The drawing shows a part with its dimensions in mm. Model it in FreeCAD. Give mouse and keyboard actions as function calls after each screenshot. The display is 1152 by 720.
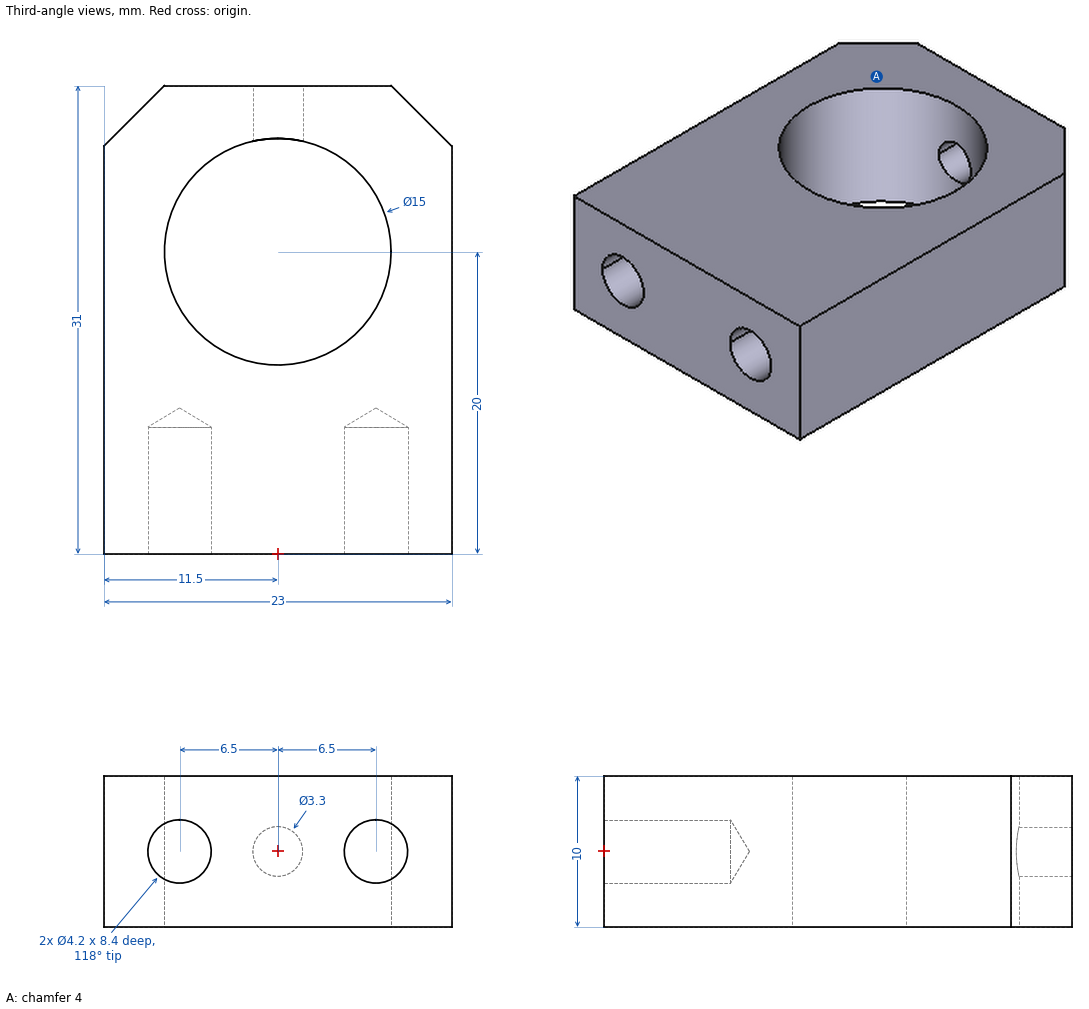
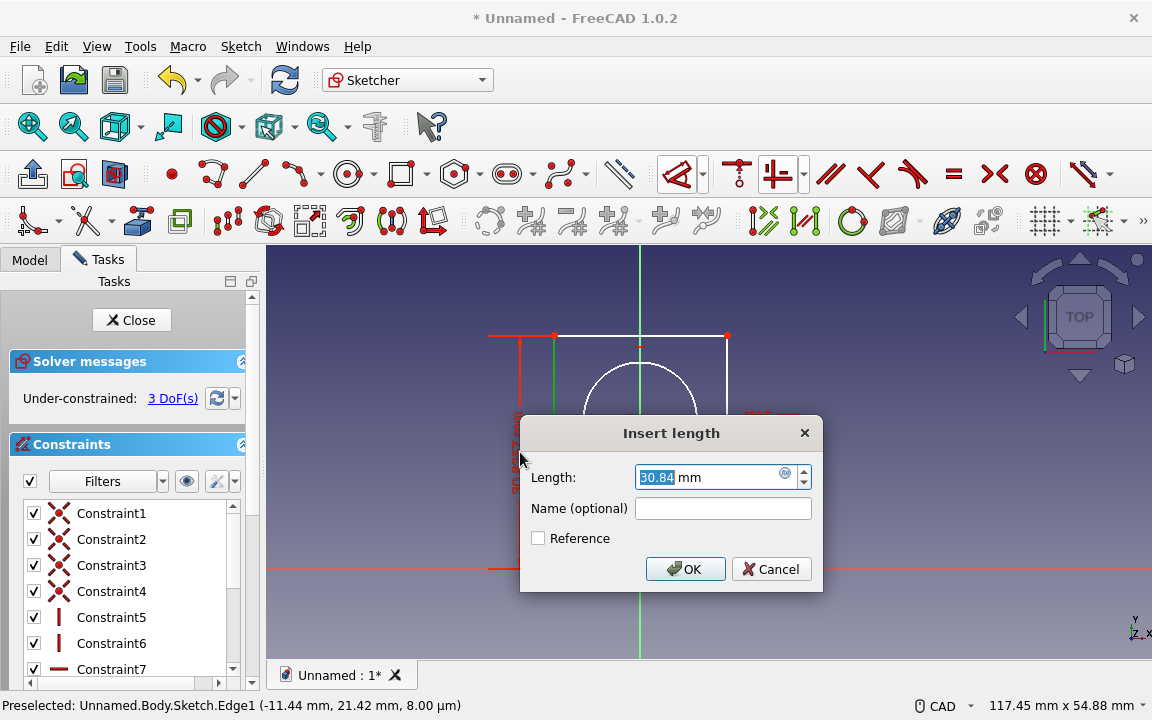
text(31)
key(Return)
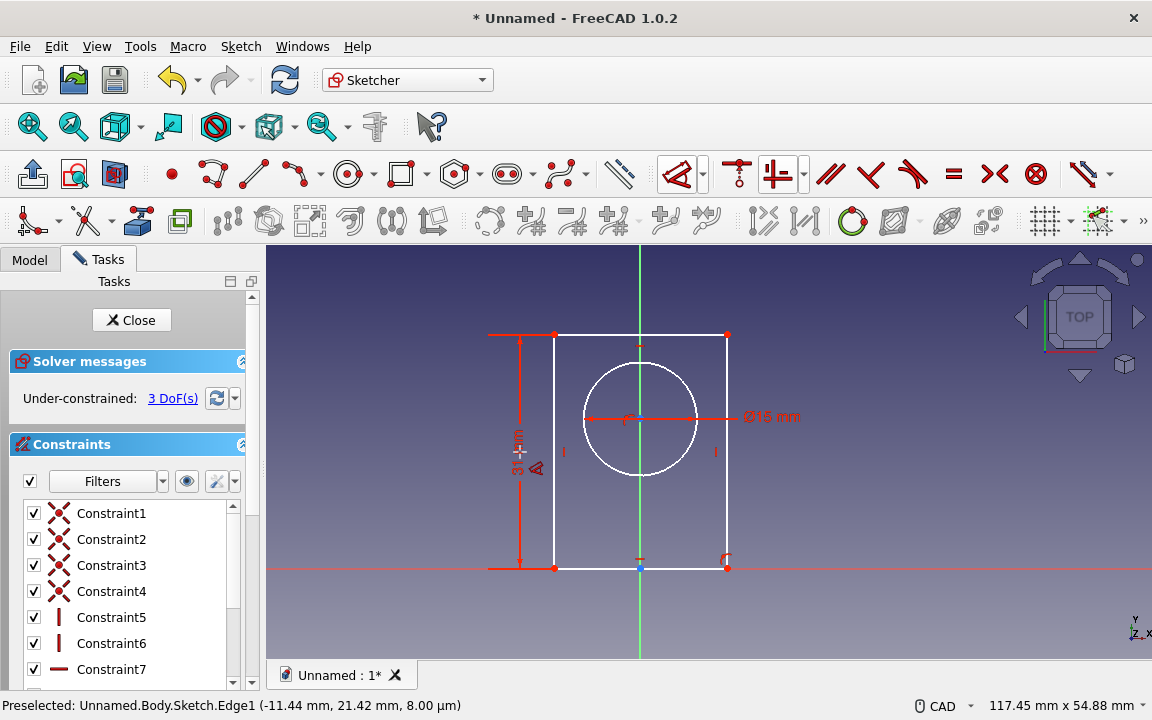
click(606, 569)
click(601, 603)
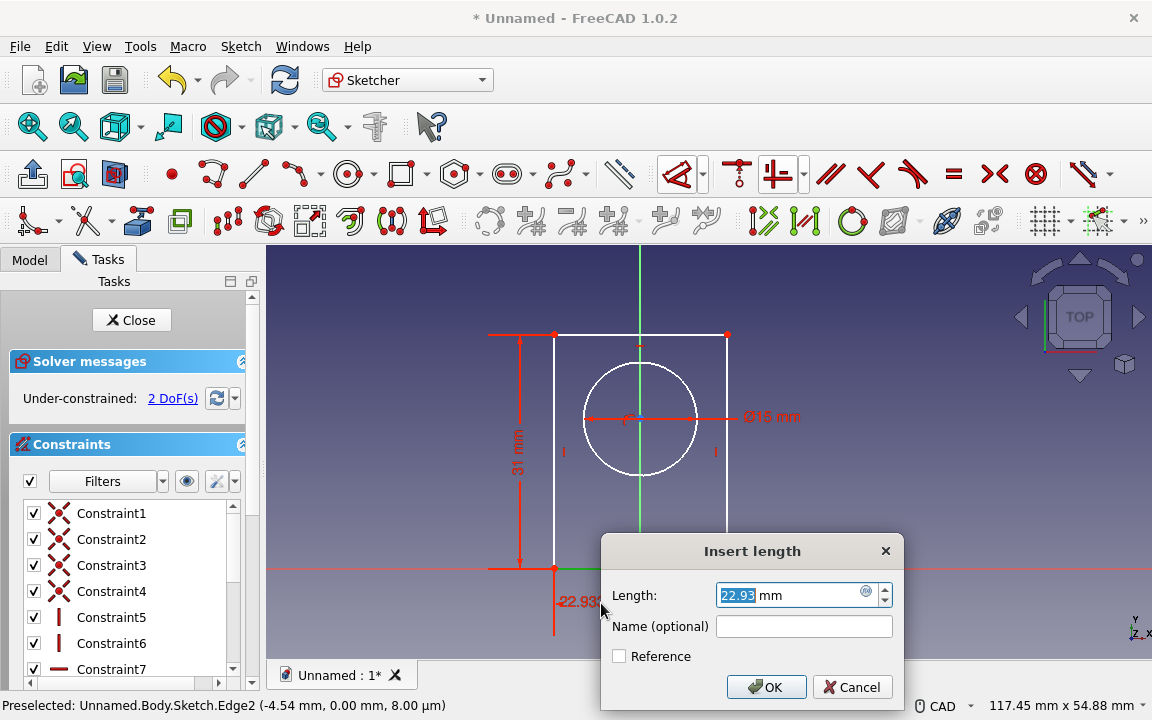
text(23)
key(Return)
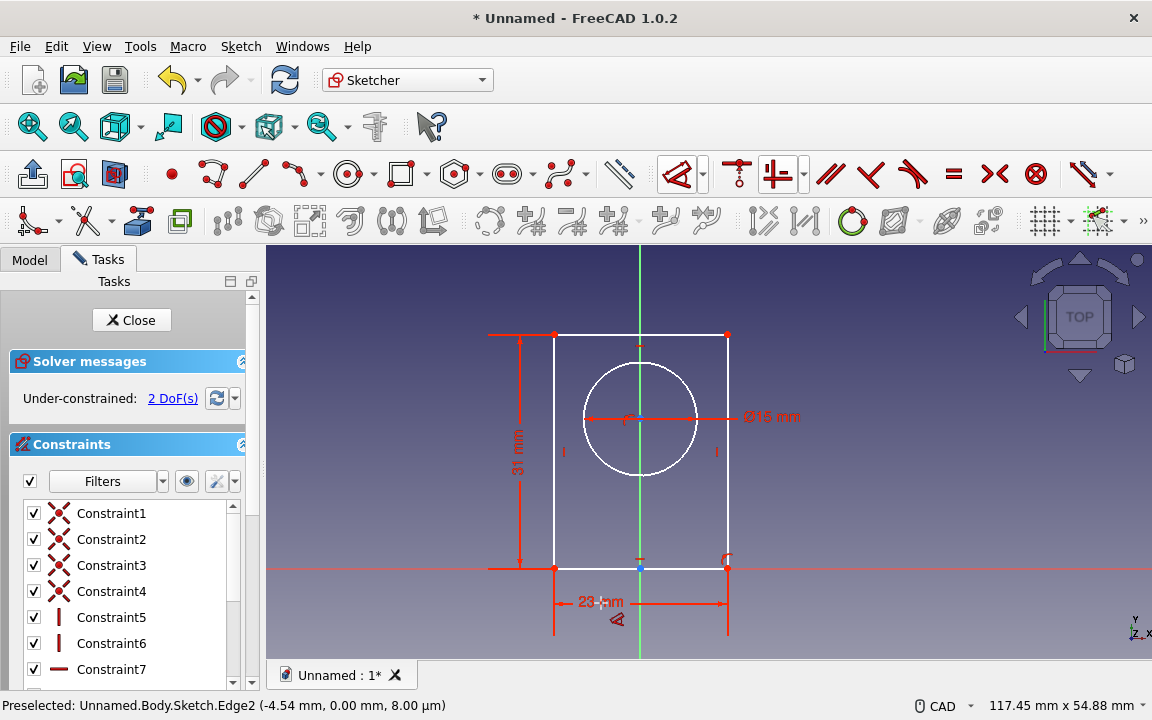
click(640, 419)
click(674, 494)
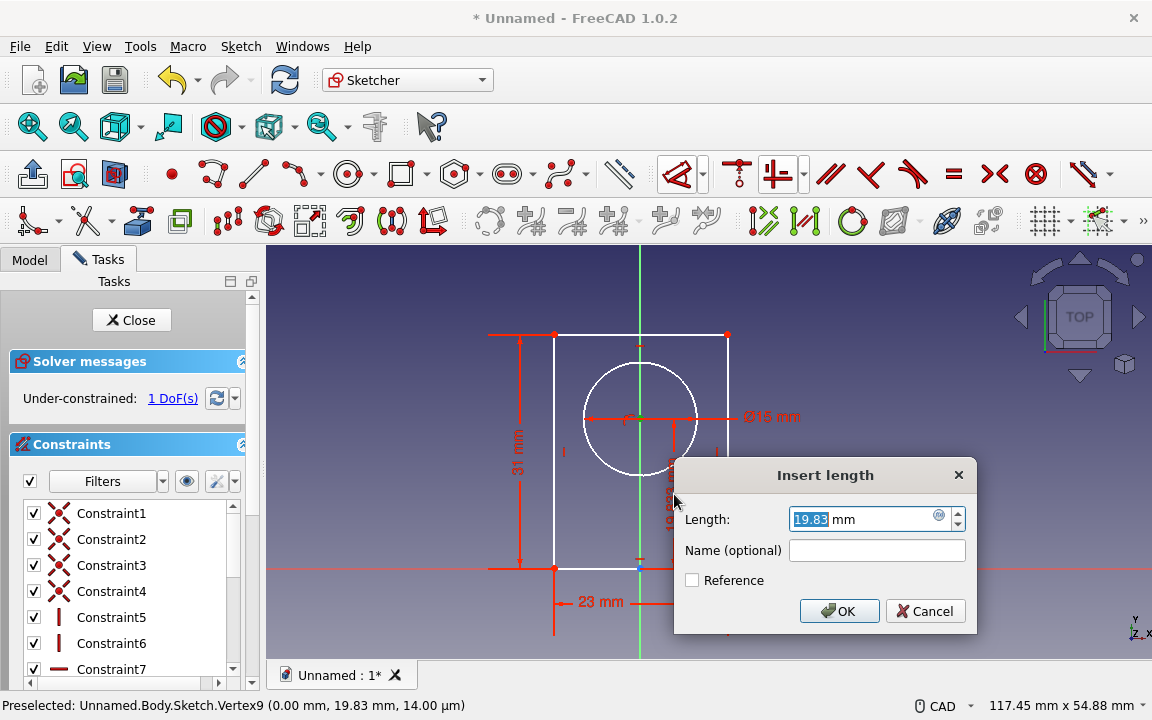
text(20)
key(Return)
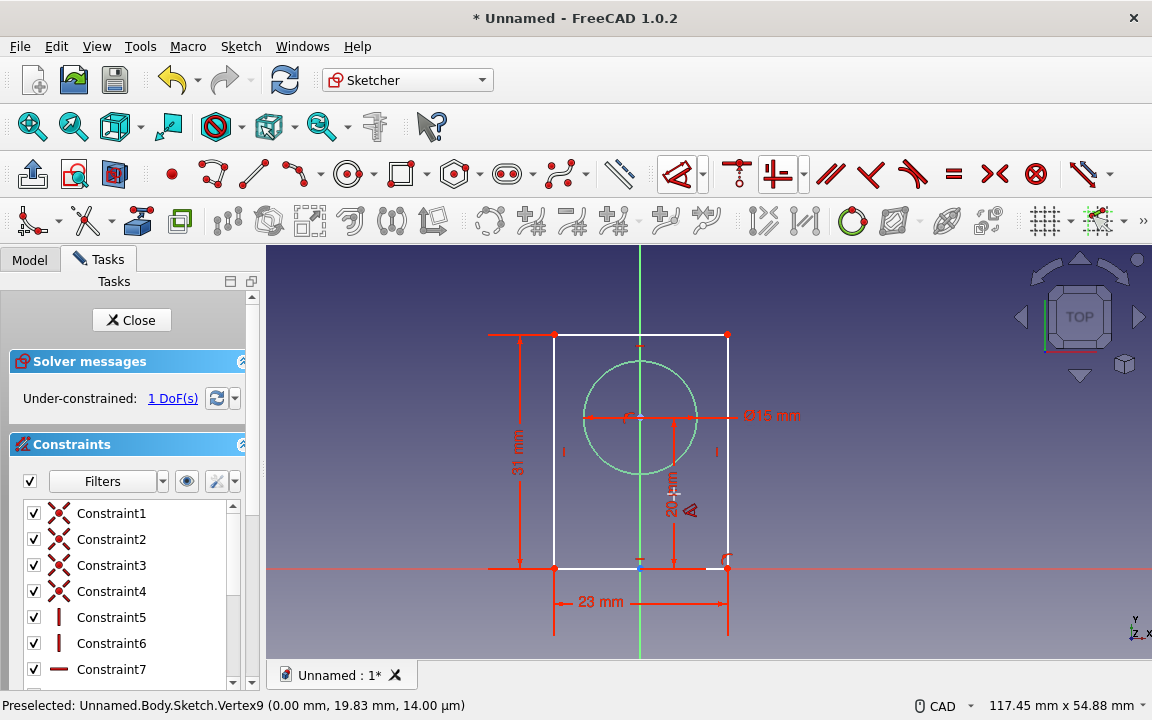
click(554, 335)
click(597, 301)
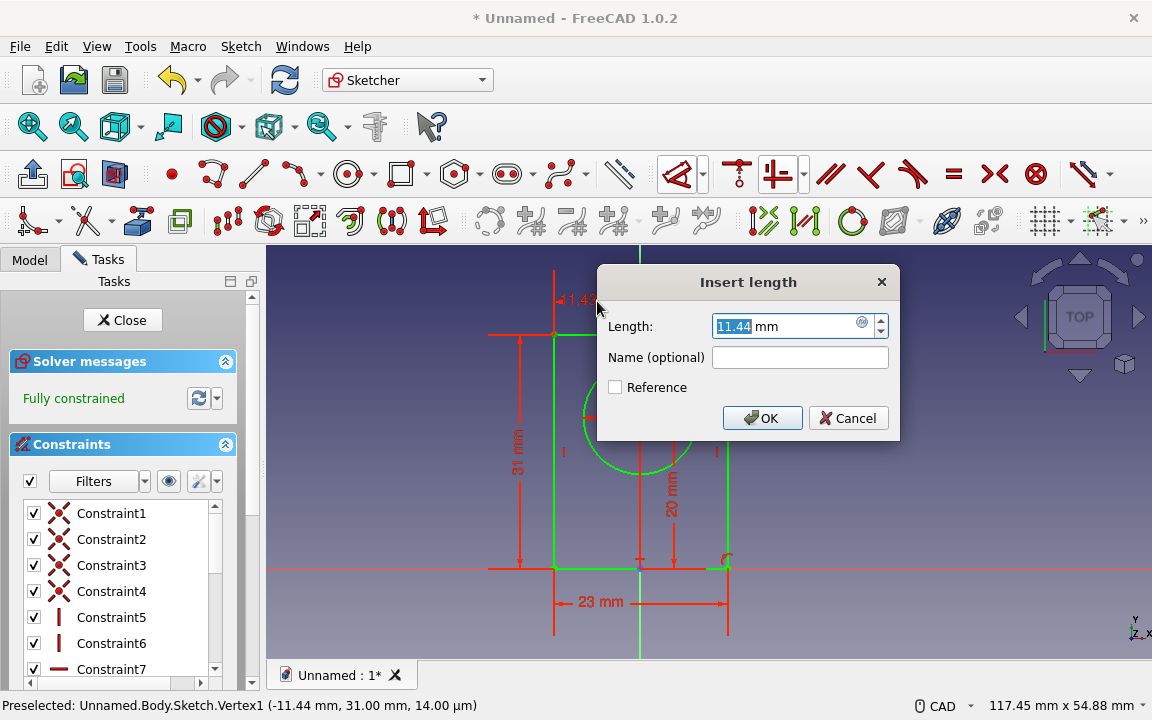
text(11.5)
key(Return)
key(Escape)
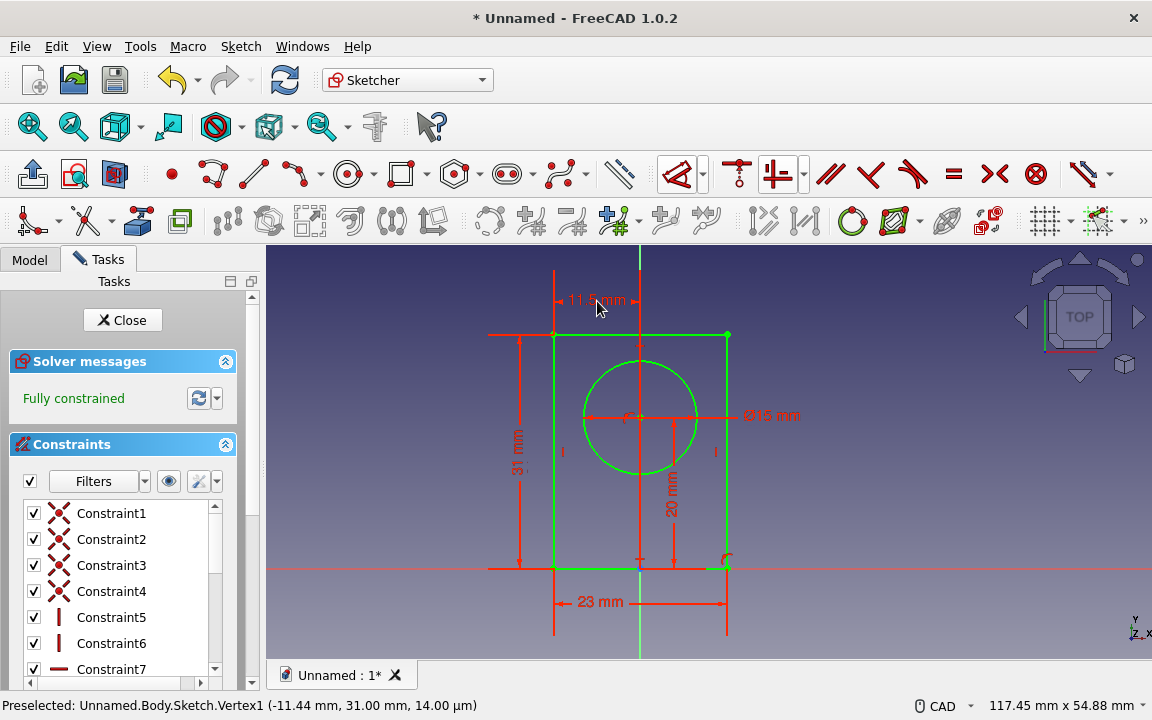
click(123, 320)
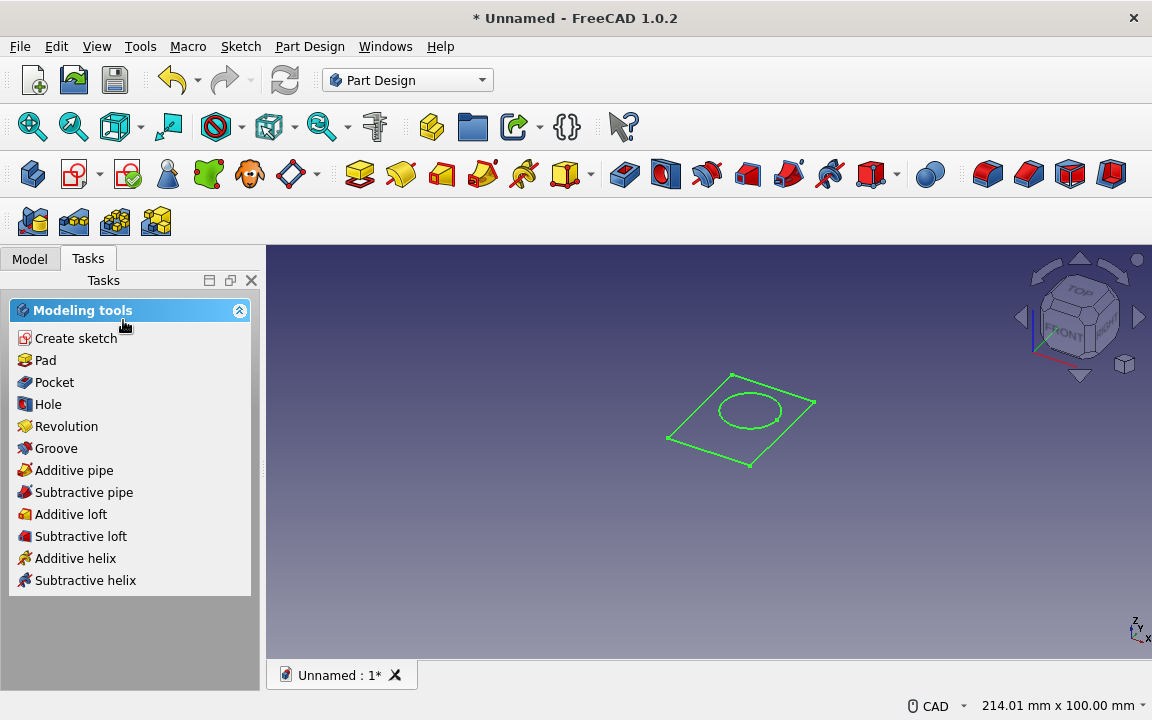
click(360, 174)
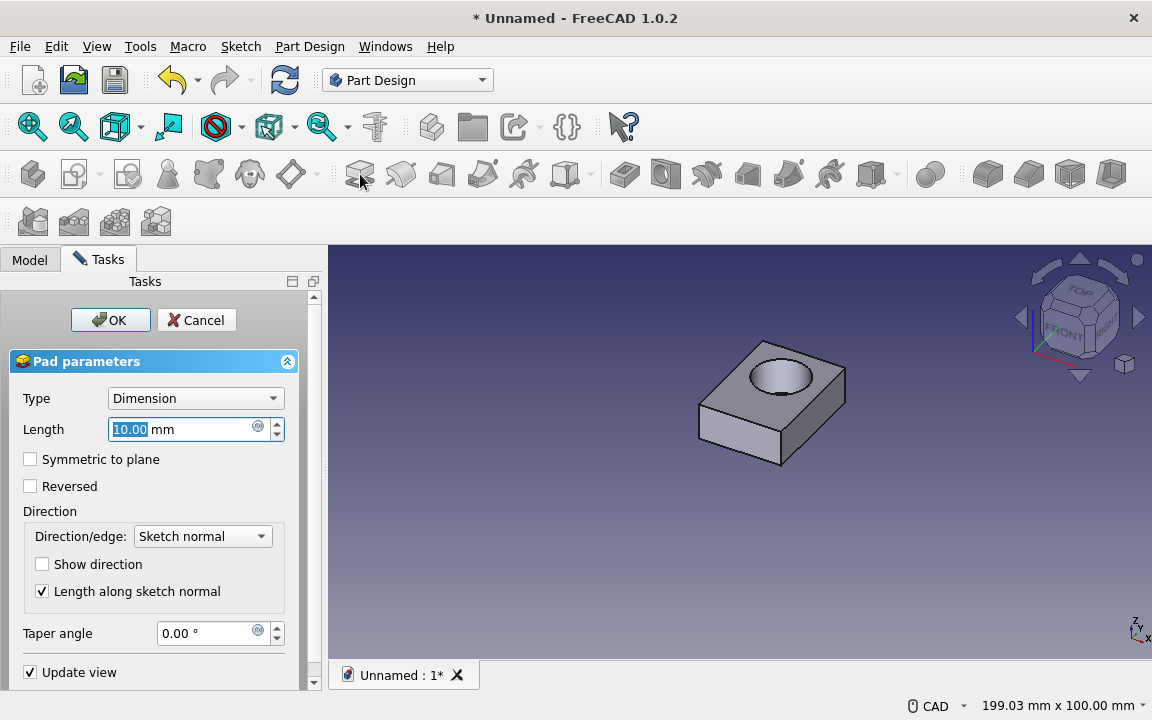
text(10)
key(Tab)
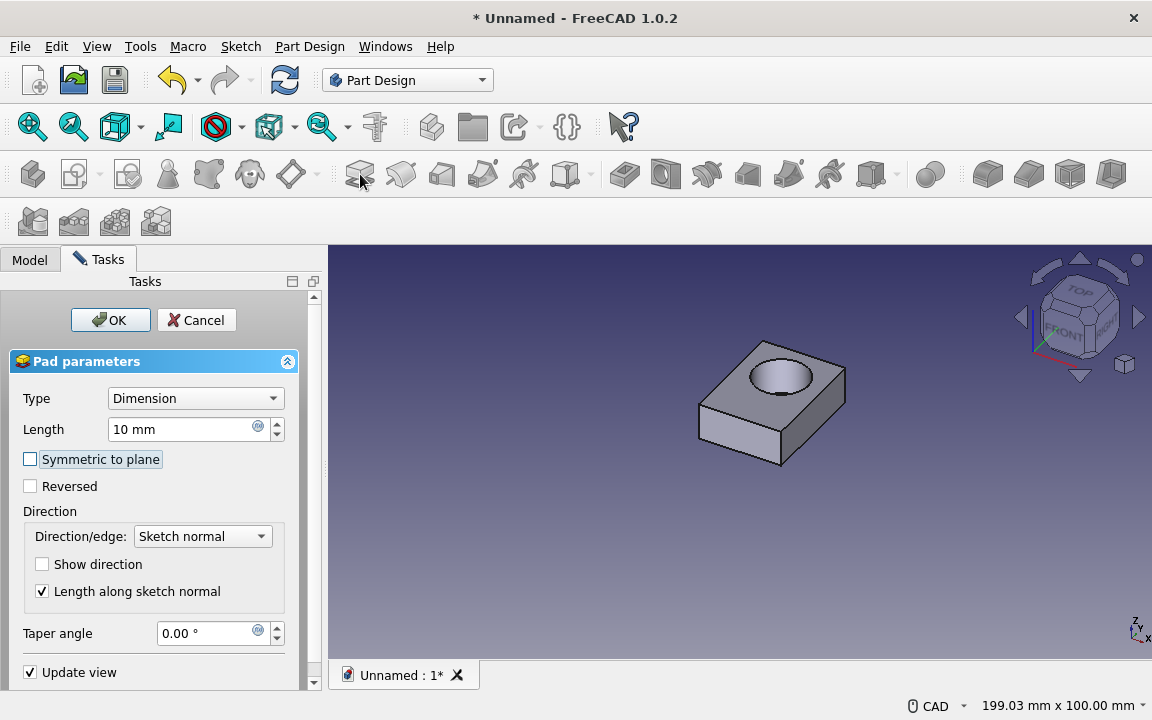
click(31, 459)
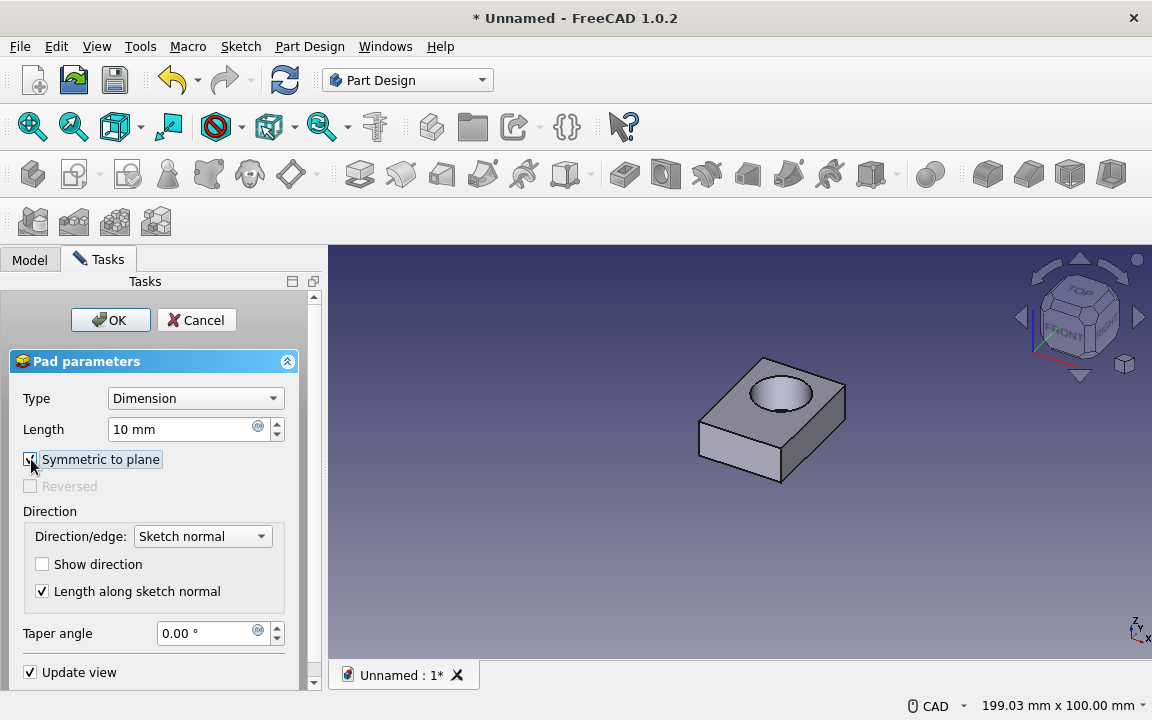
click(111, 320)